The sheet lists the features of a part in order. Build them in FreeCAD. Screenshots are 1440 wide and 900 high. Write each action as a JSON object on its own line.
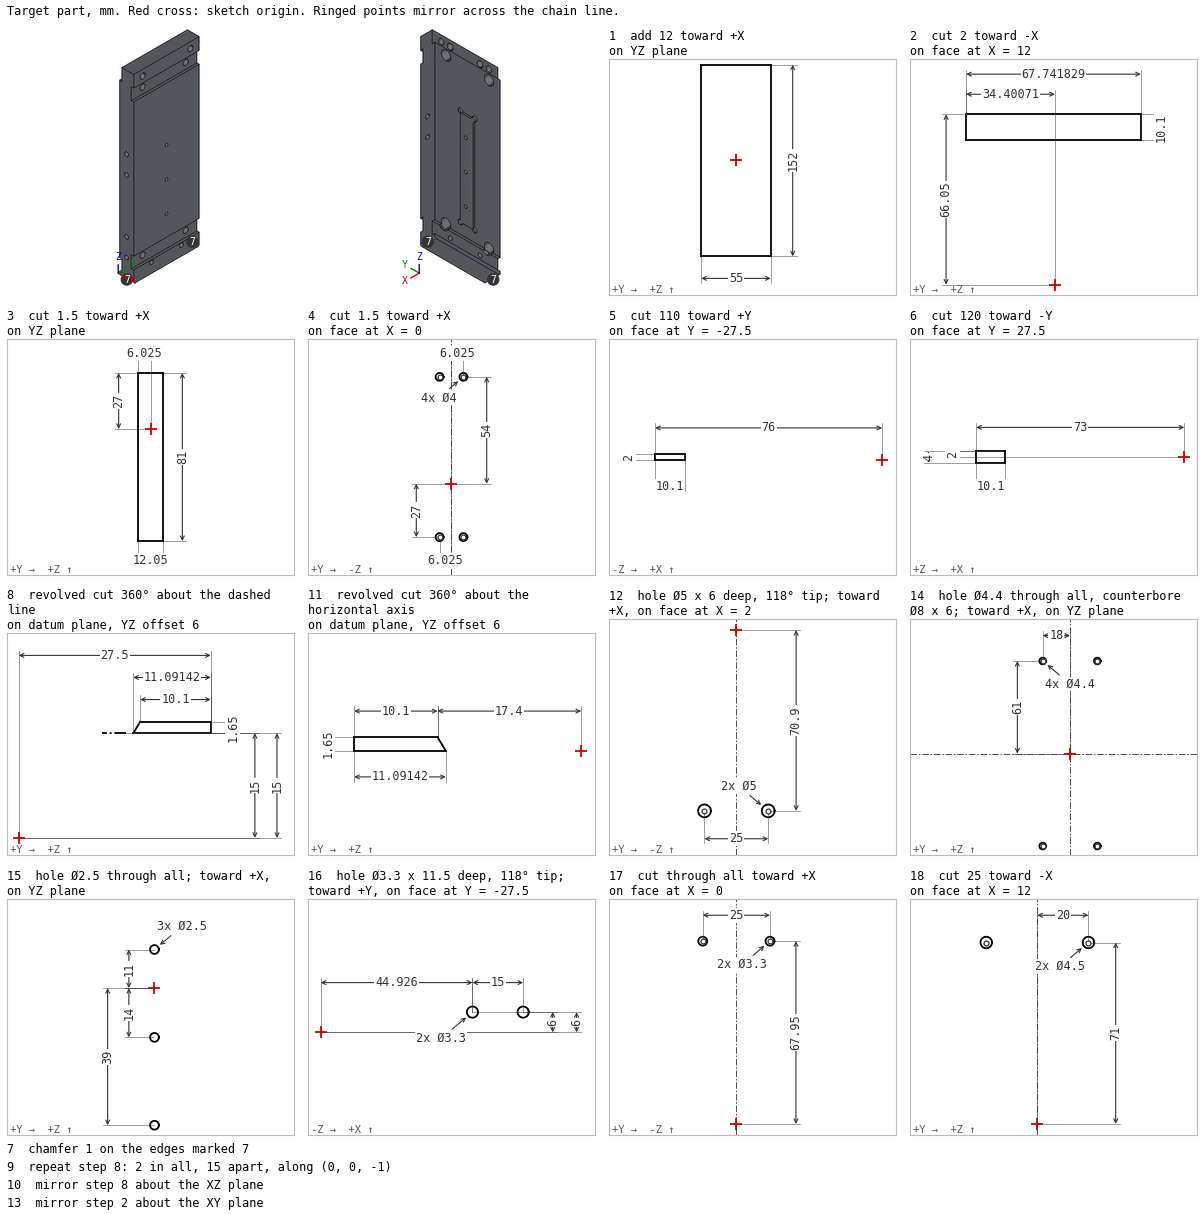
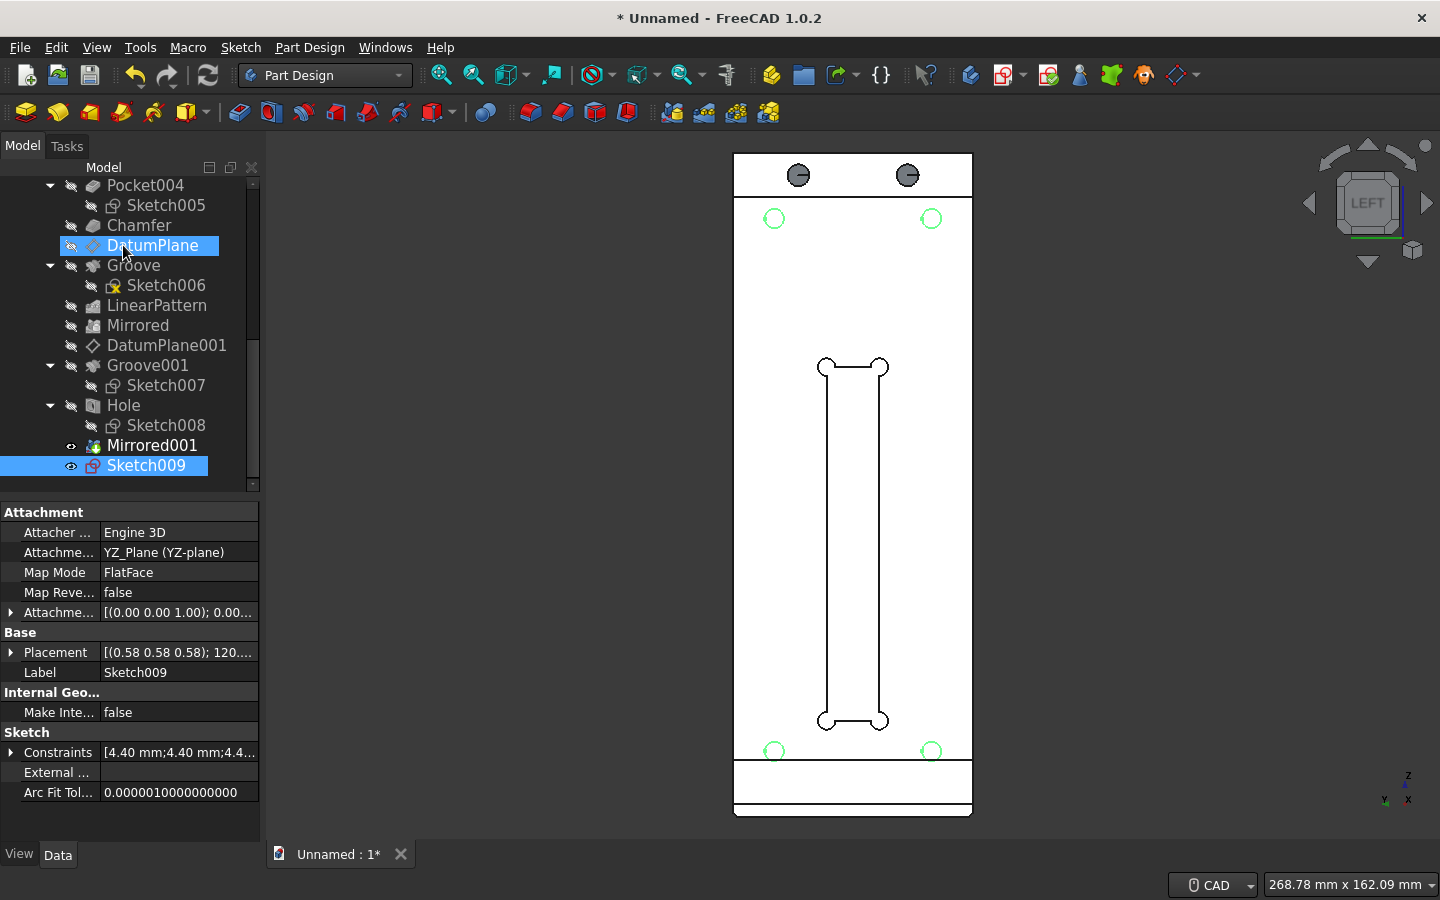
{"action": "left_click", "coordinate": [272, 112]}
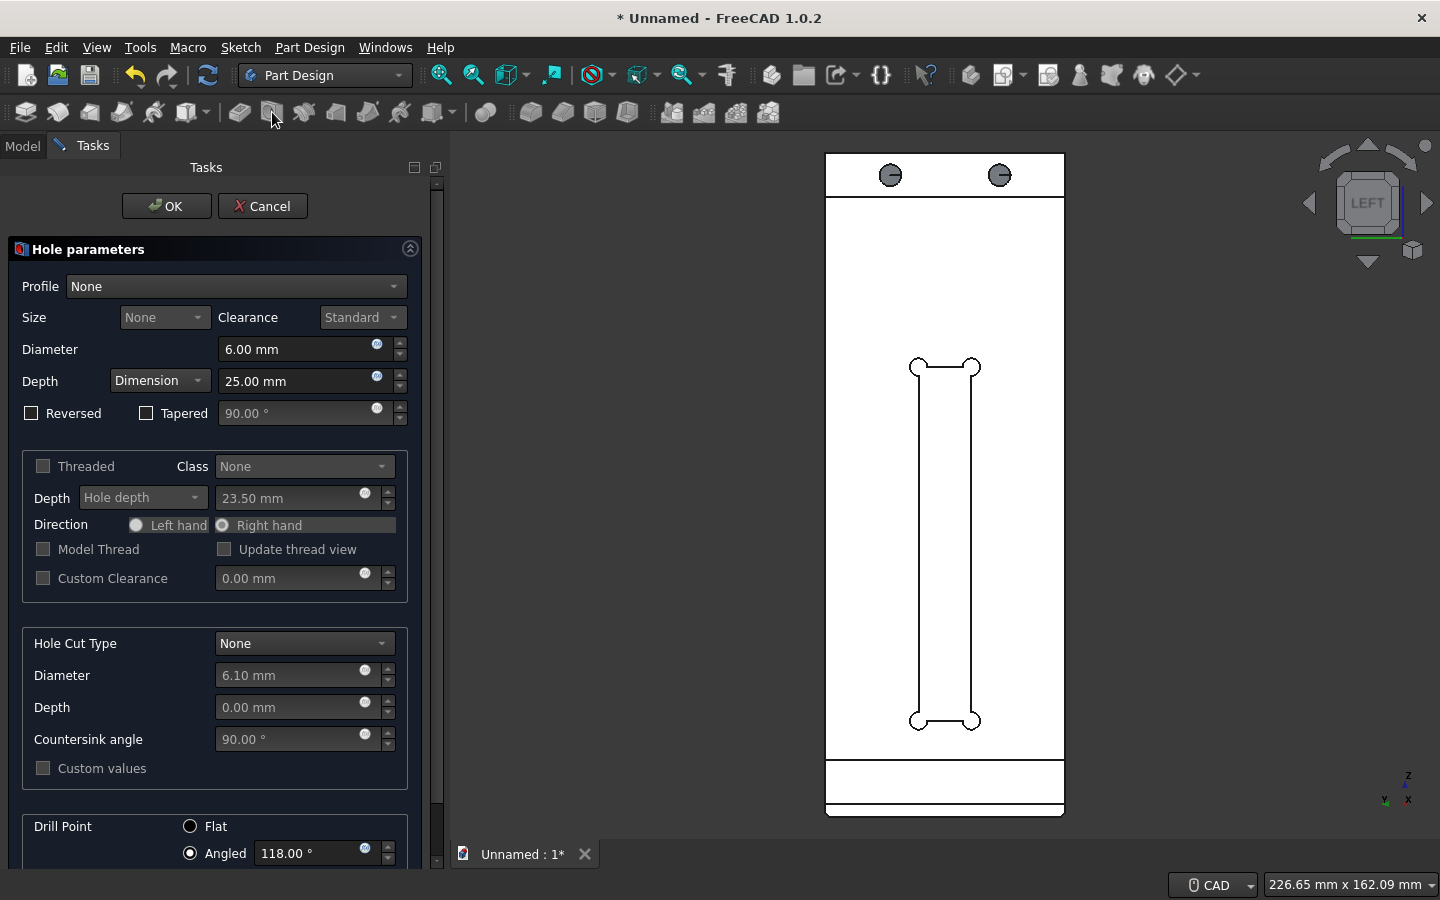
{"action": "triple_click", "coordinate": [305, 349]}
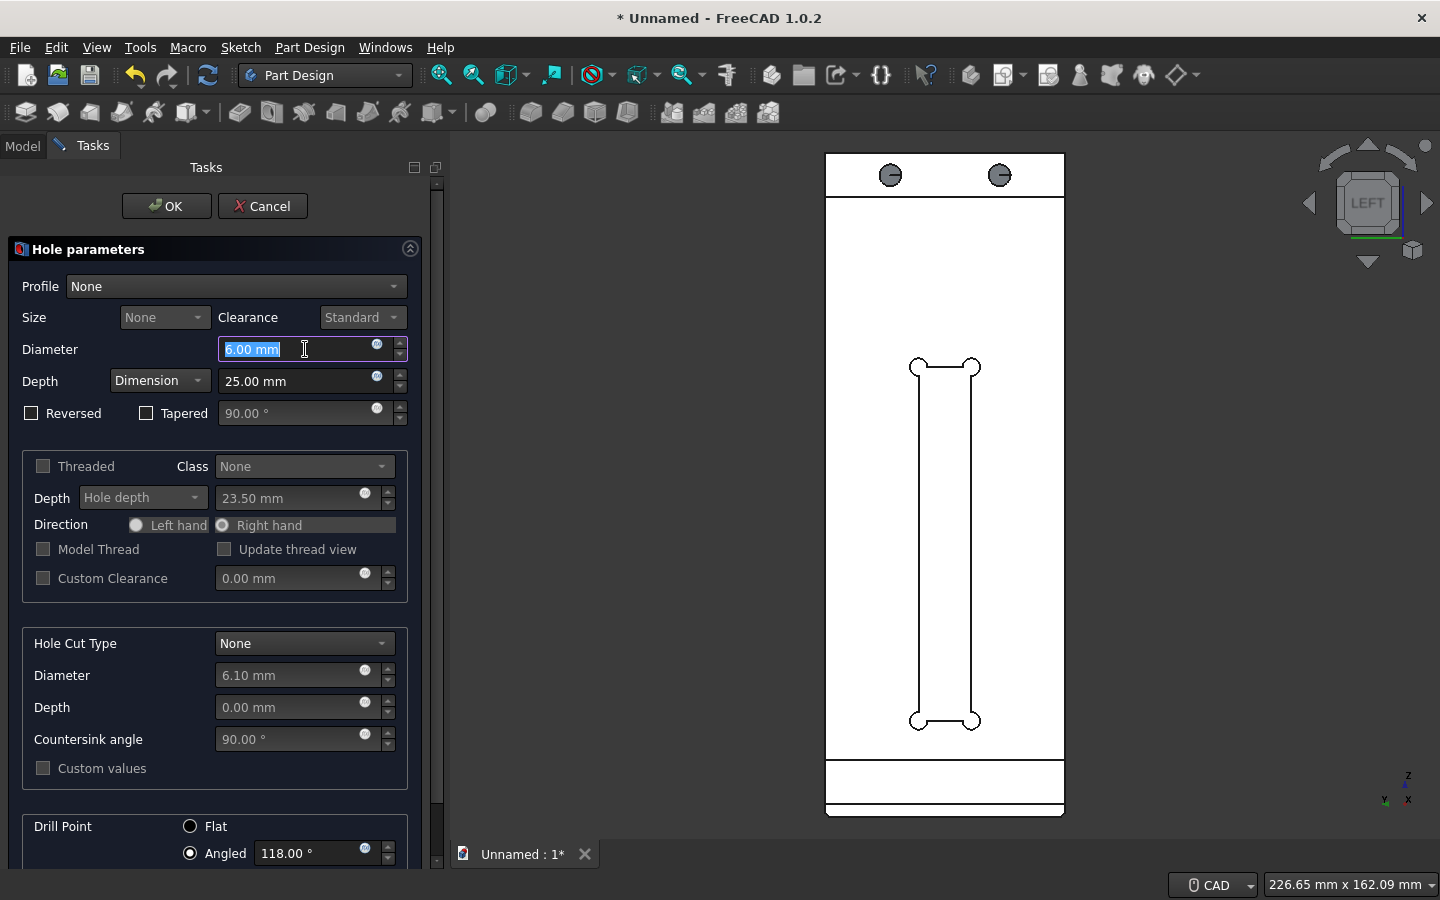
{"action": "type", "text": "4.4"}
{"action": "key", "text": "Tab"}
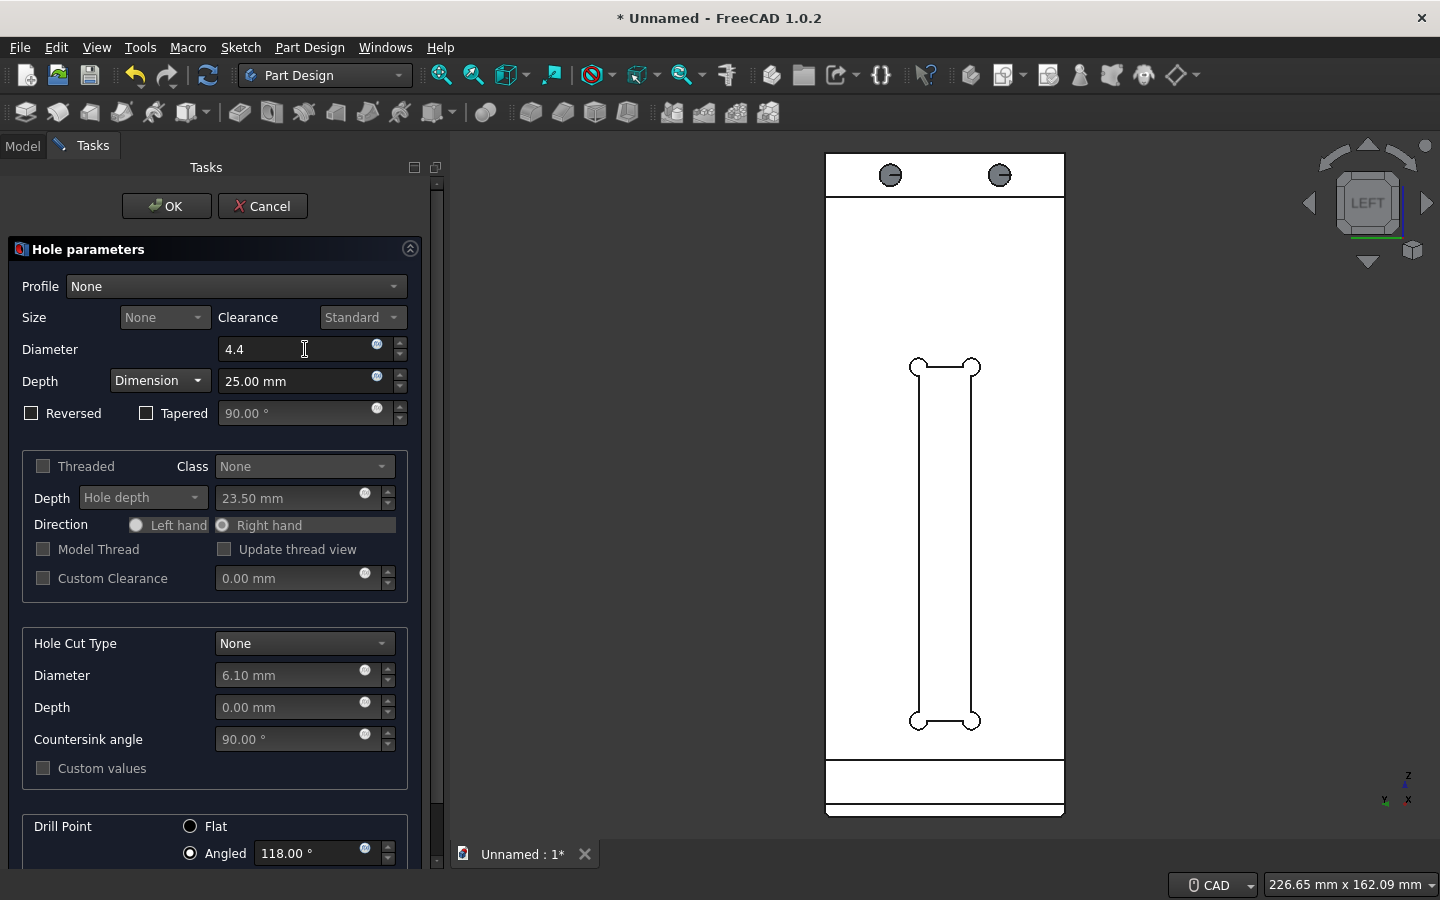
{"action": "left_click", "coordinate": [161, 380]}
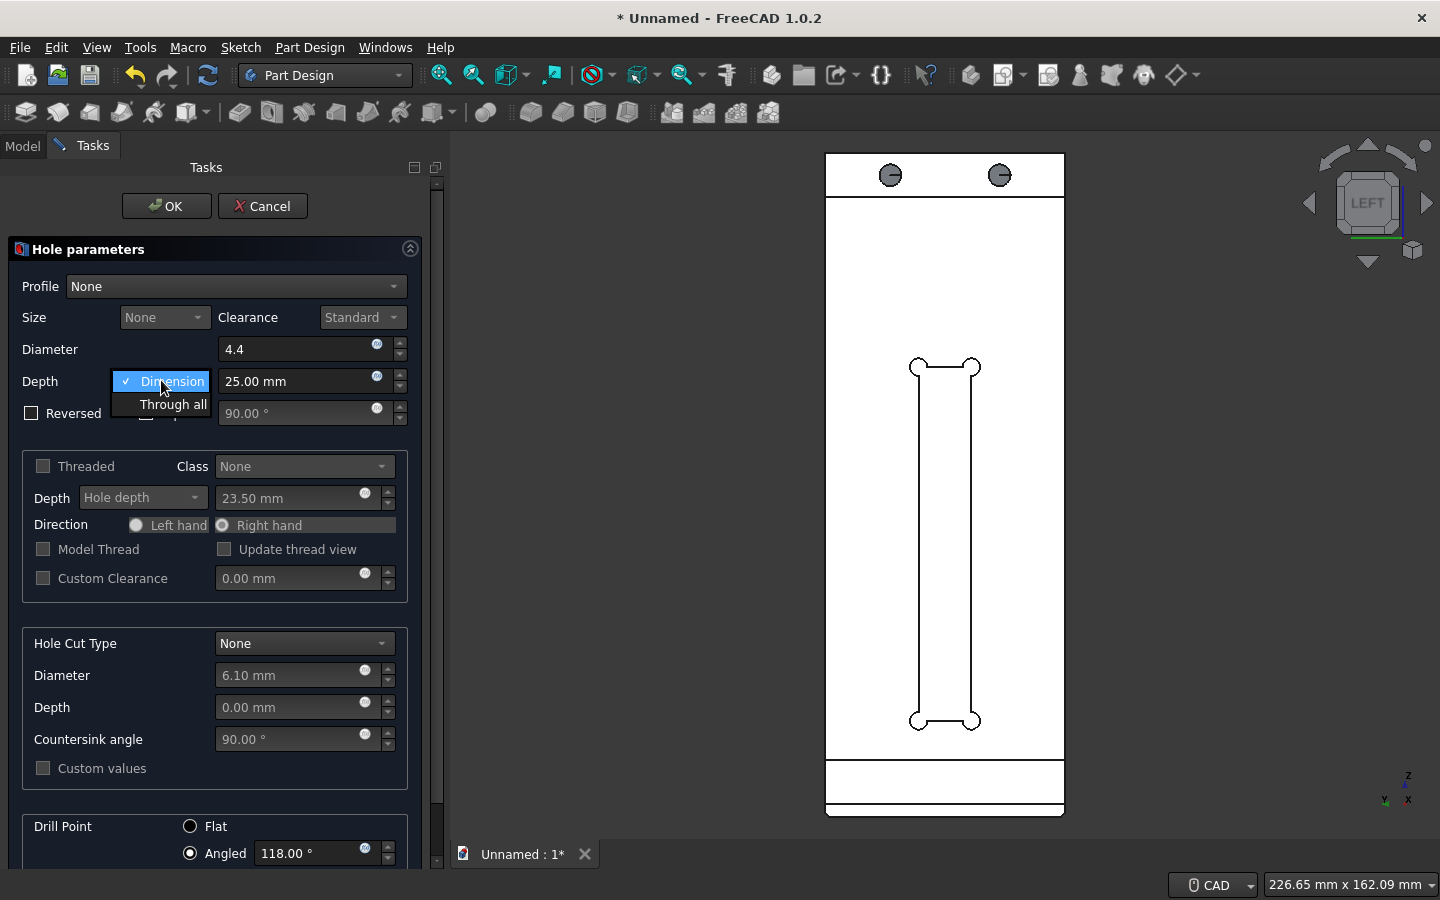
{"action": "left_click", "coordinate": [160, 404]}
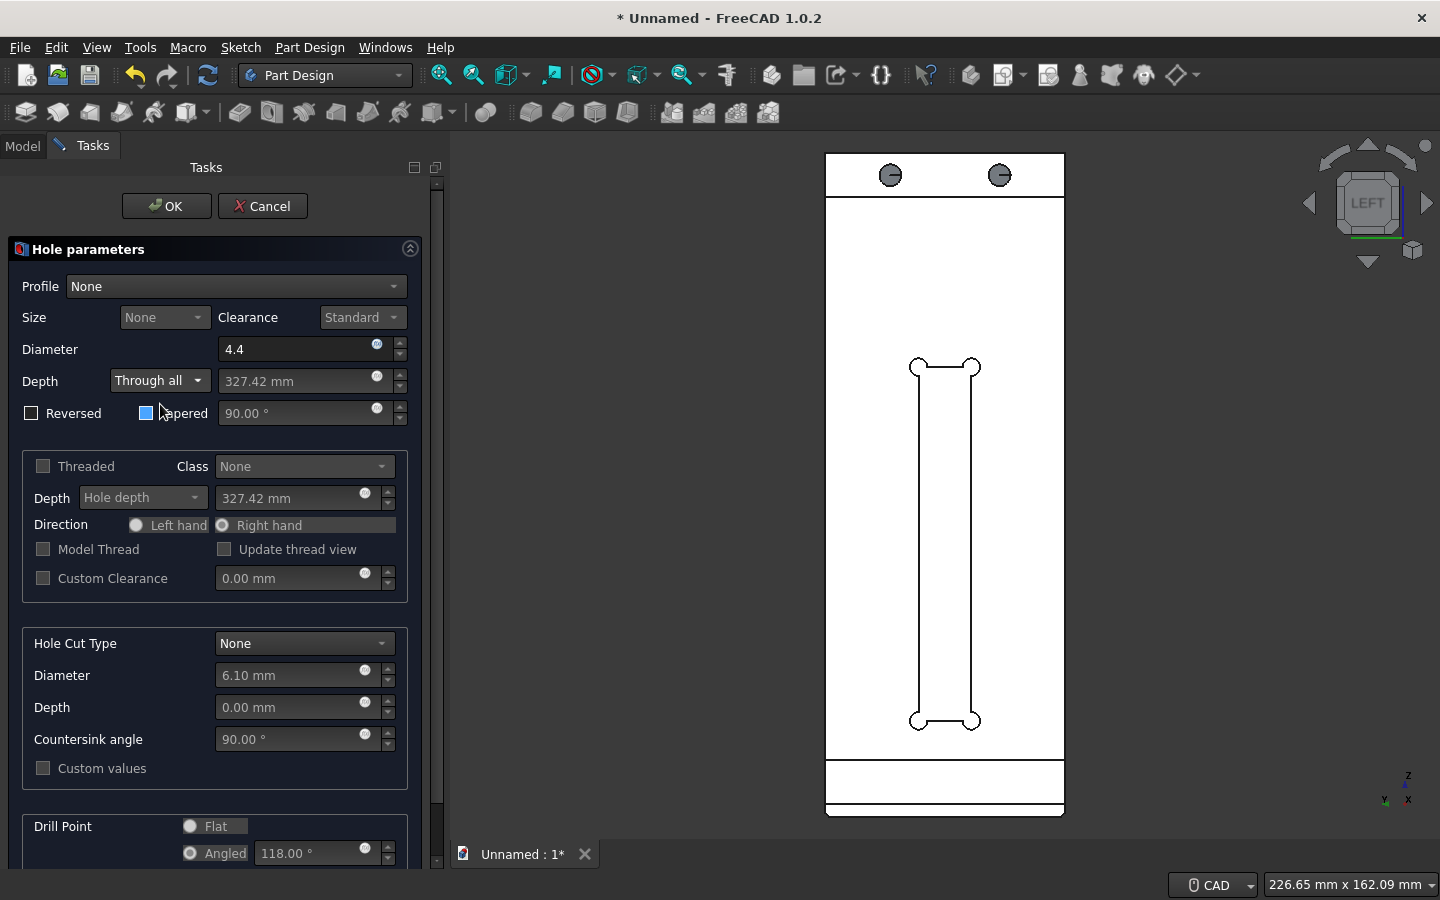
{"action": "left_click", "coordinate": [30, 413]}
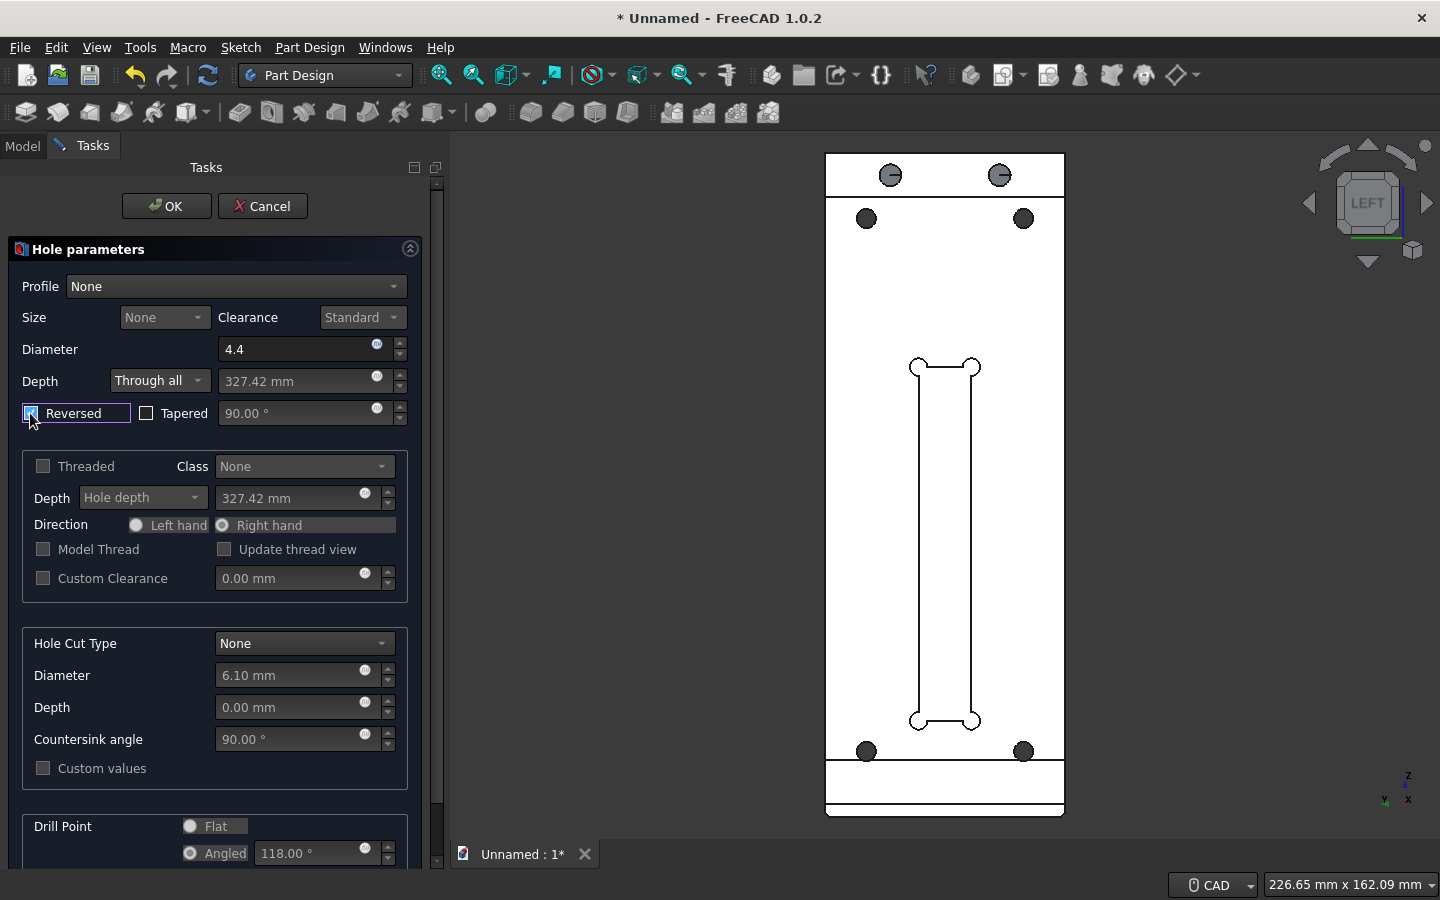
{"action": "left_click", "coordinate": [306, 644]}